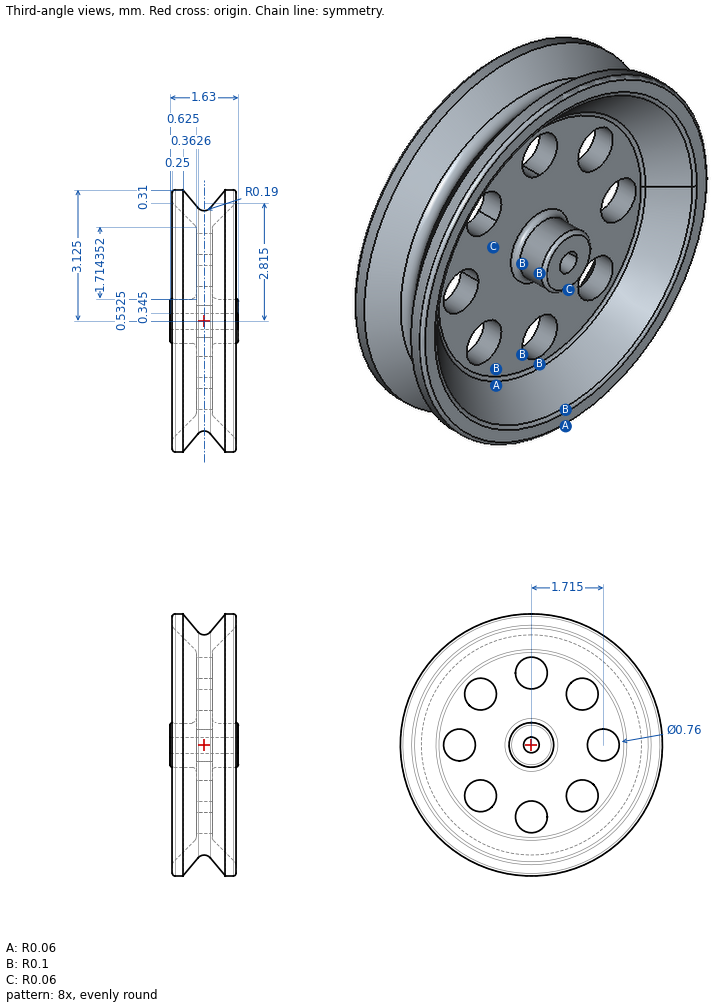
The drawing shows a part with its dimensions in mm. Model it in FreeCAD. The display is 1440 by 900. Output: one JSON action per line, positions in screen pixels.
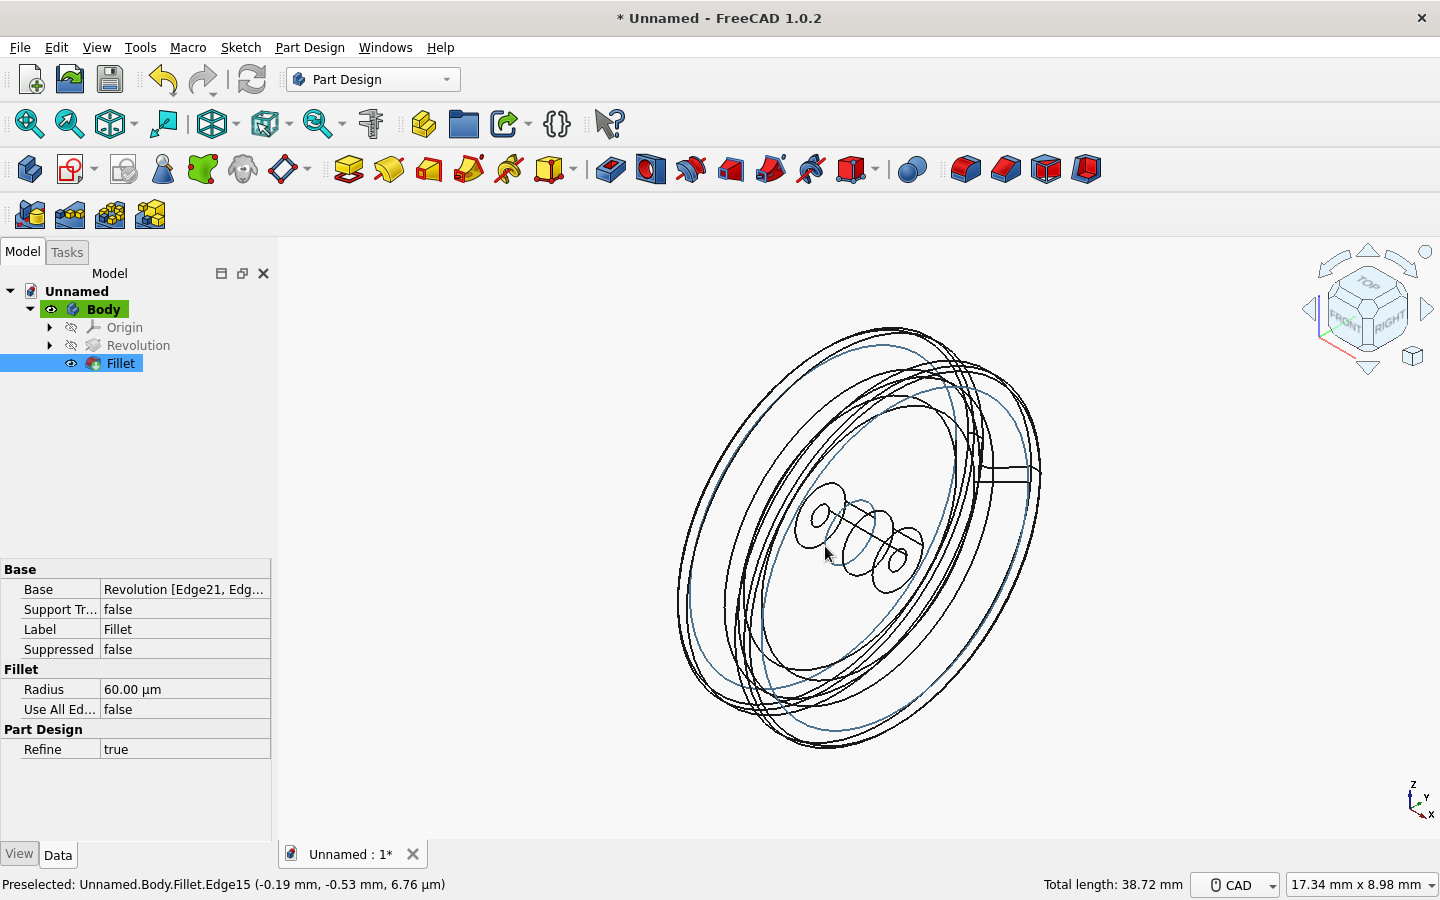
{"action": "left_click", "coordinate": [817, 668], "text": "ctrl"}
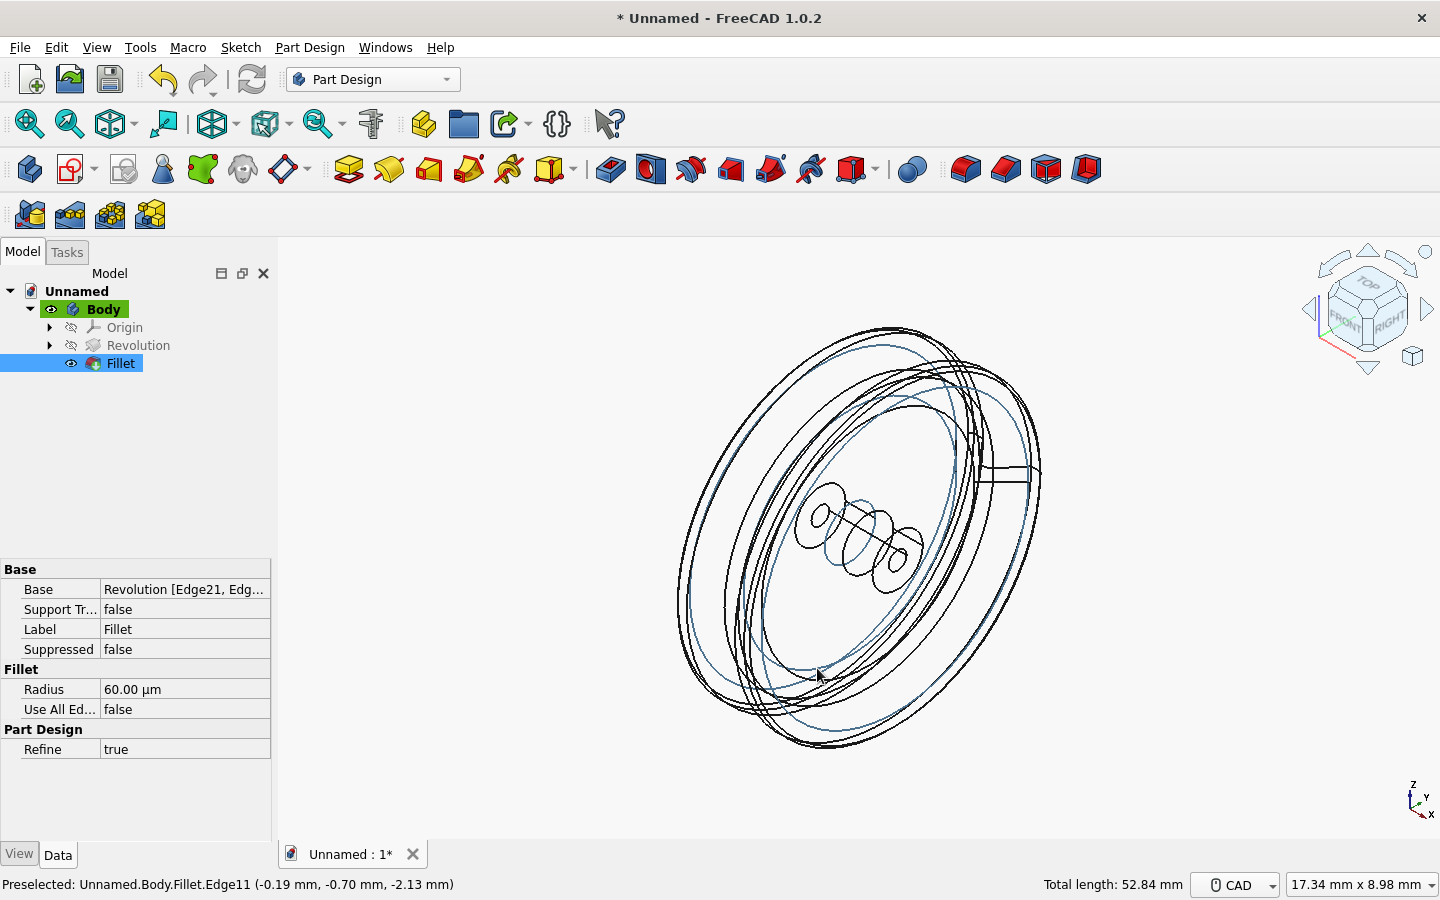
{"action": "left_click", "coordinate": [782, 664], "text": "ctrl"}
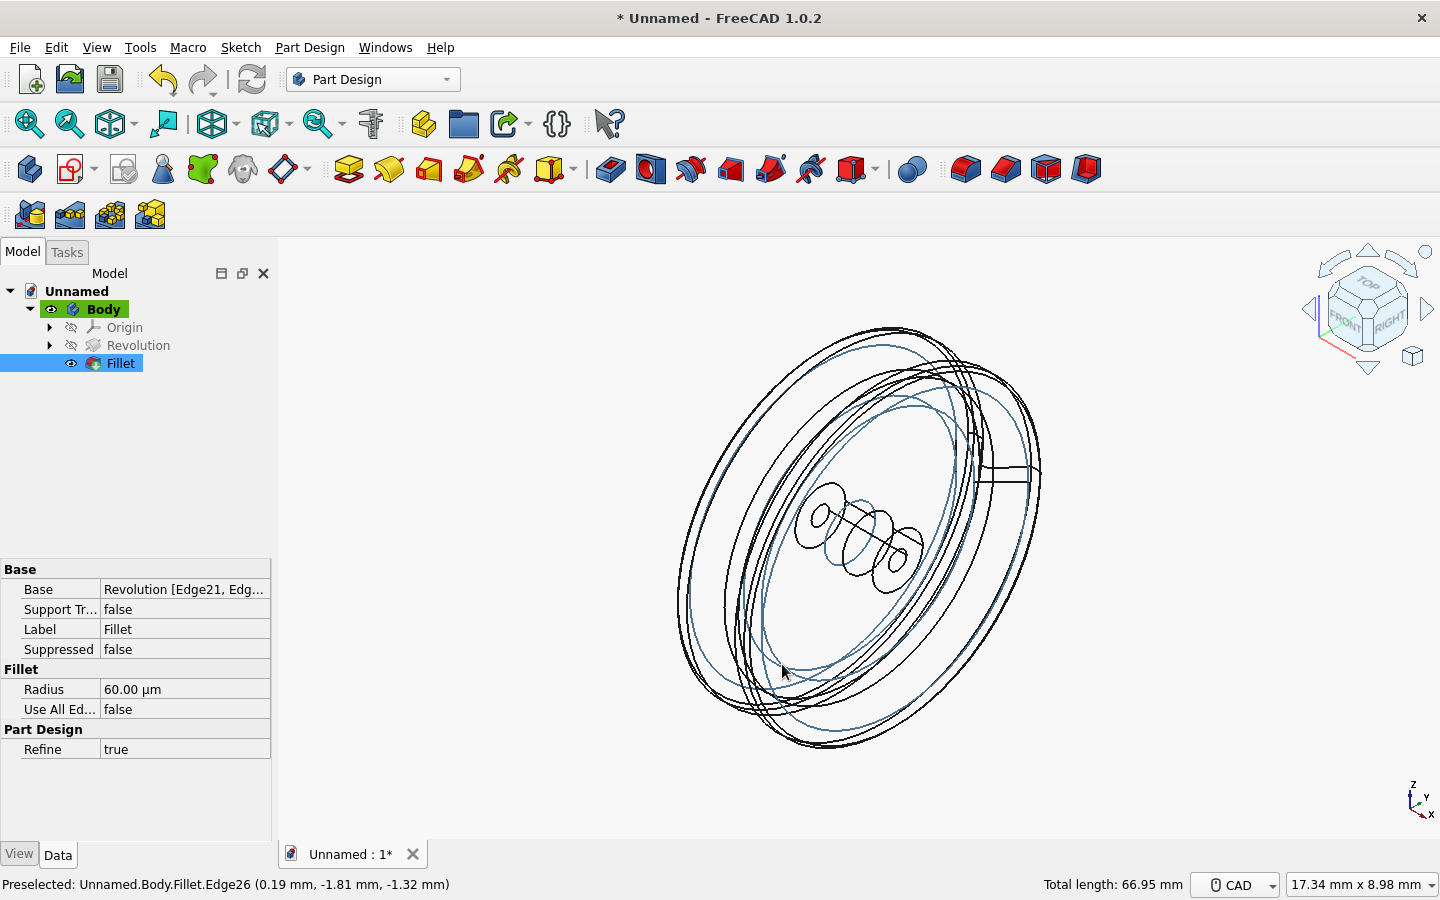
{"action": "left_click", "coordinate": [843, 557], "text": "ctrl"}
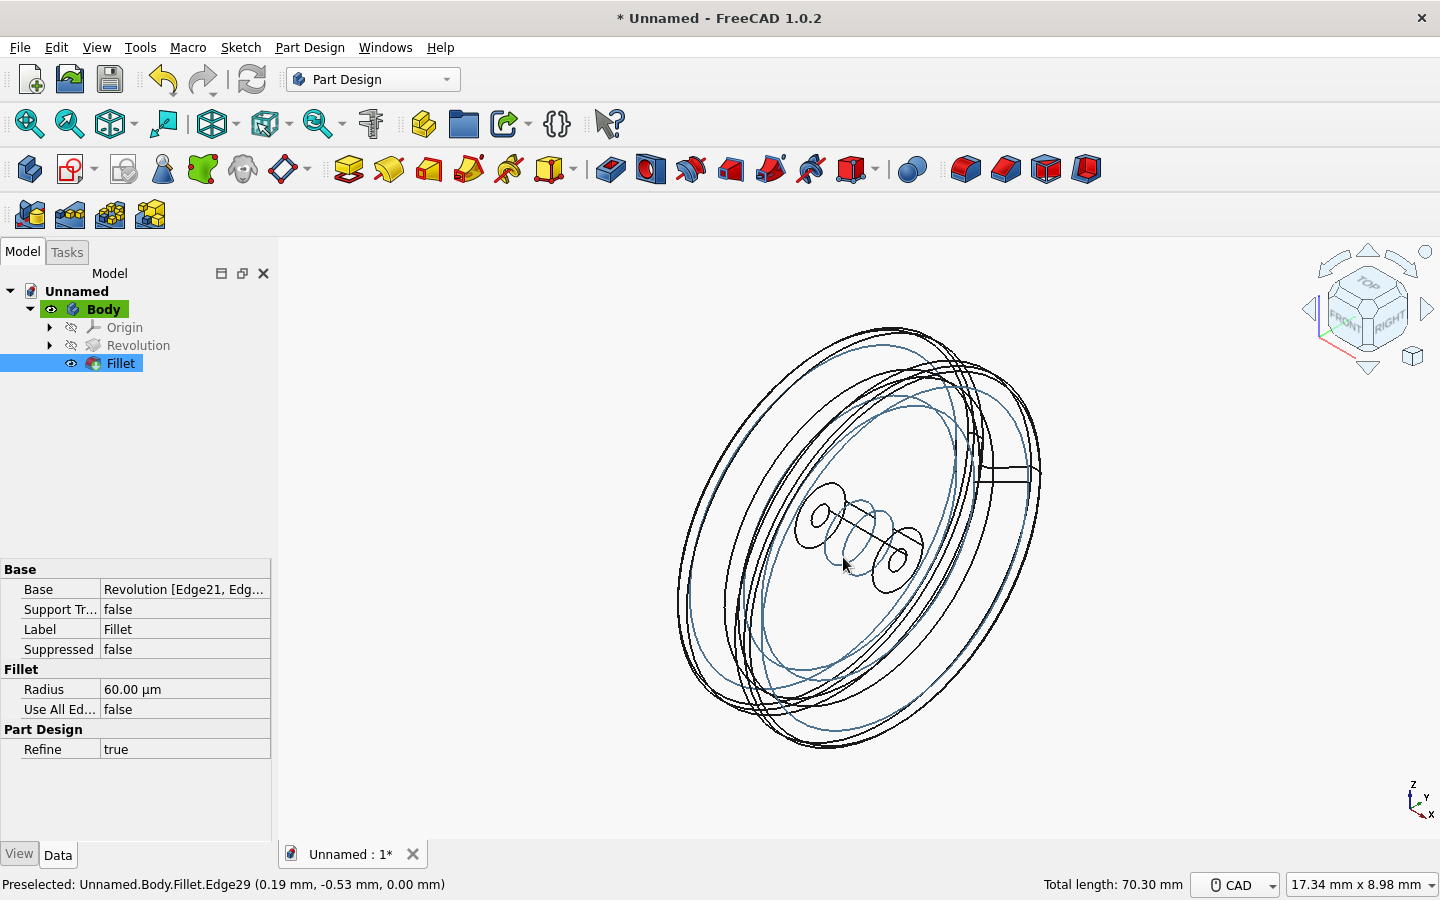
{"action": "key", "text": "v 1"}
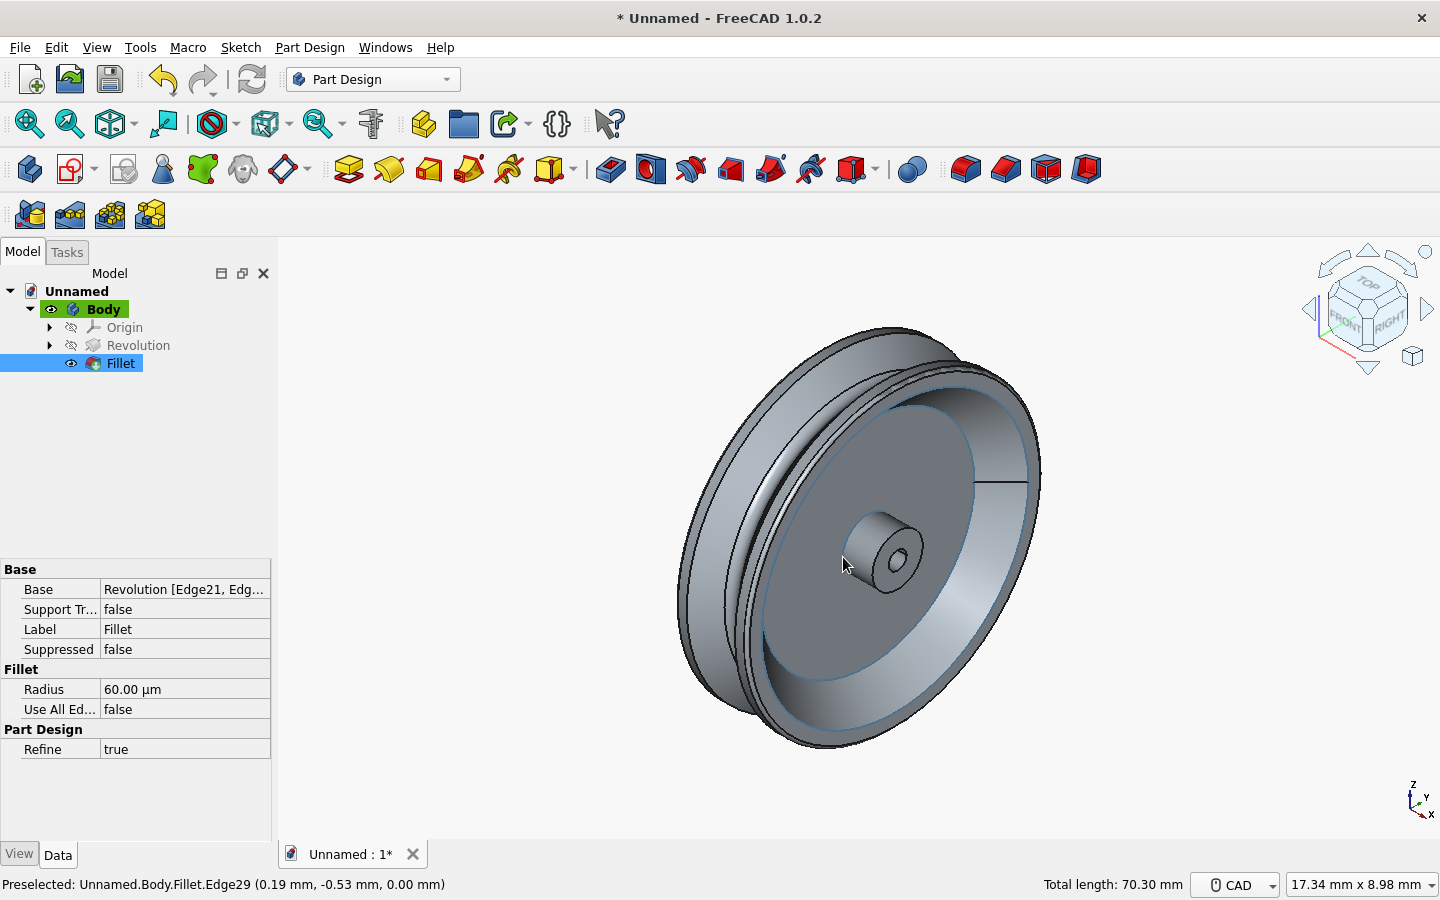
{"action": "left_click", "coordinate": [966, 170]}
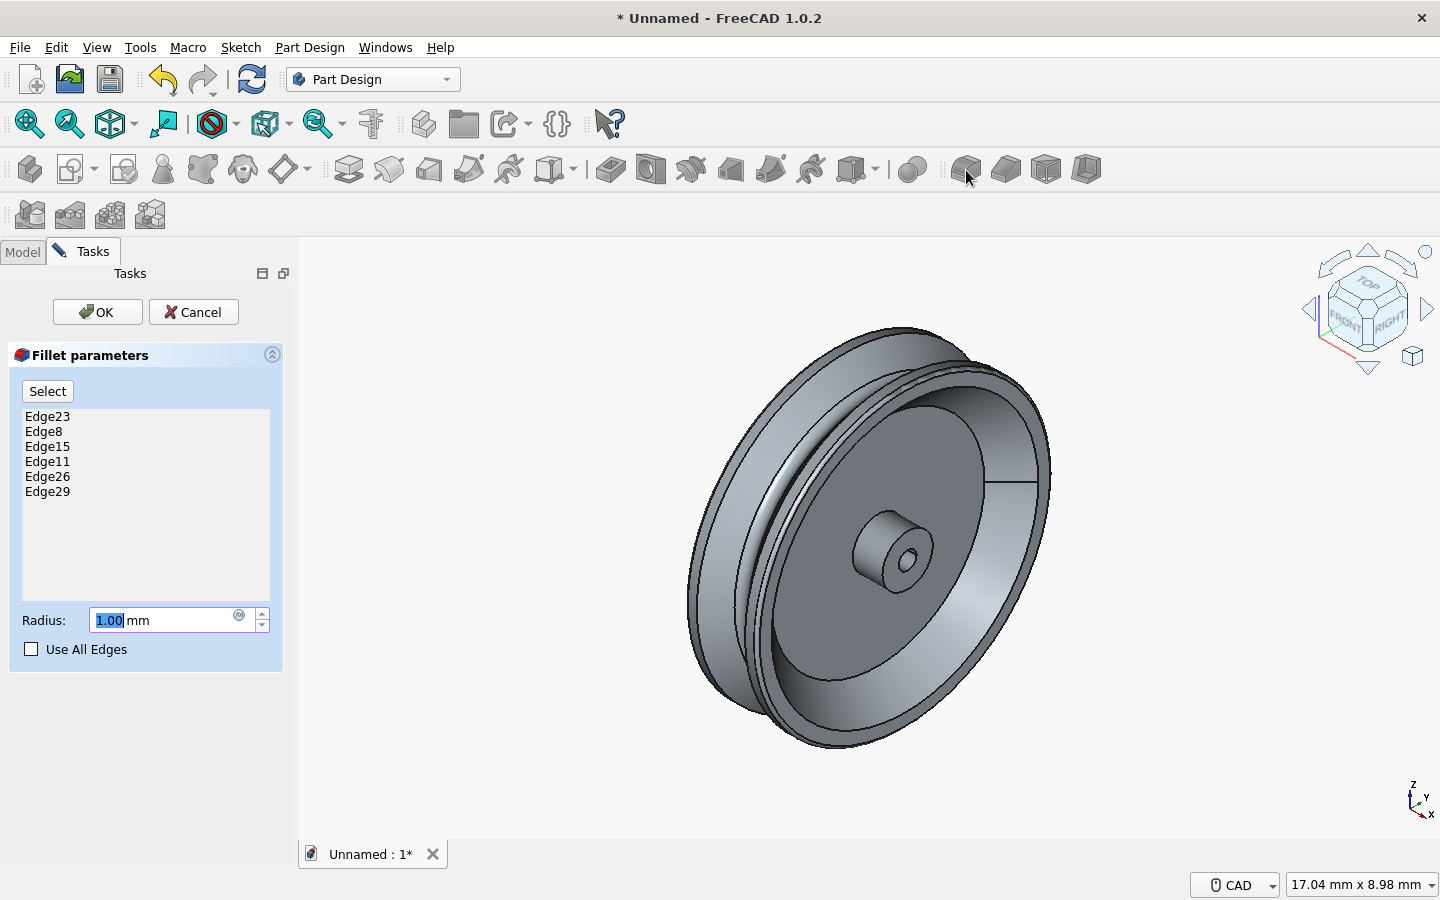
{"action": "type", "text": "0.1"}
{"action": "key", "text": "Tab"}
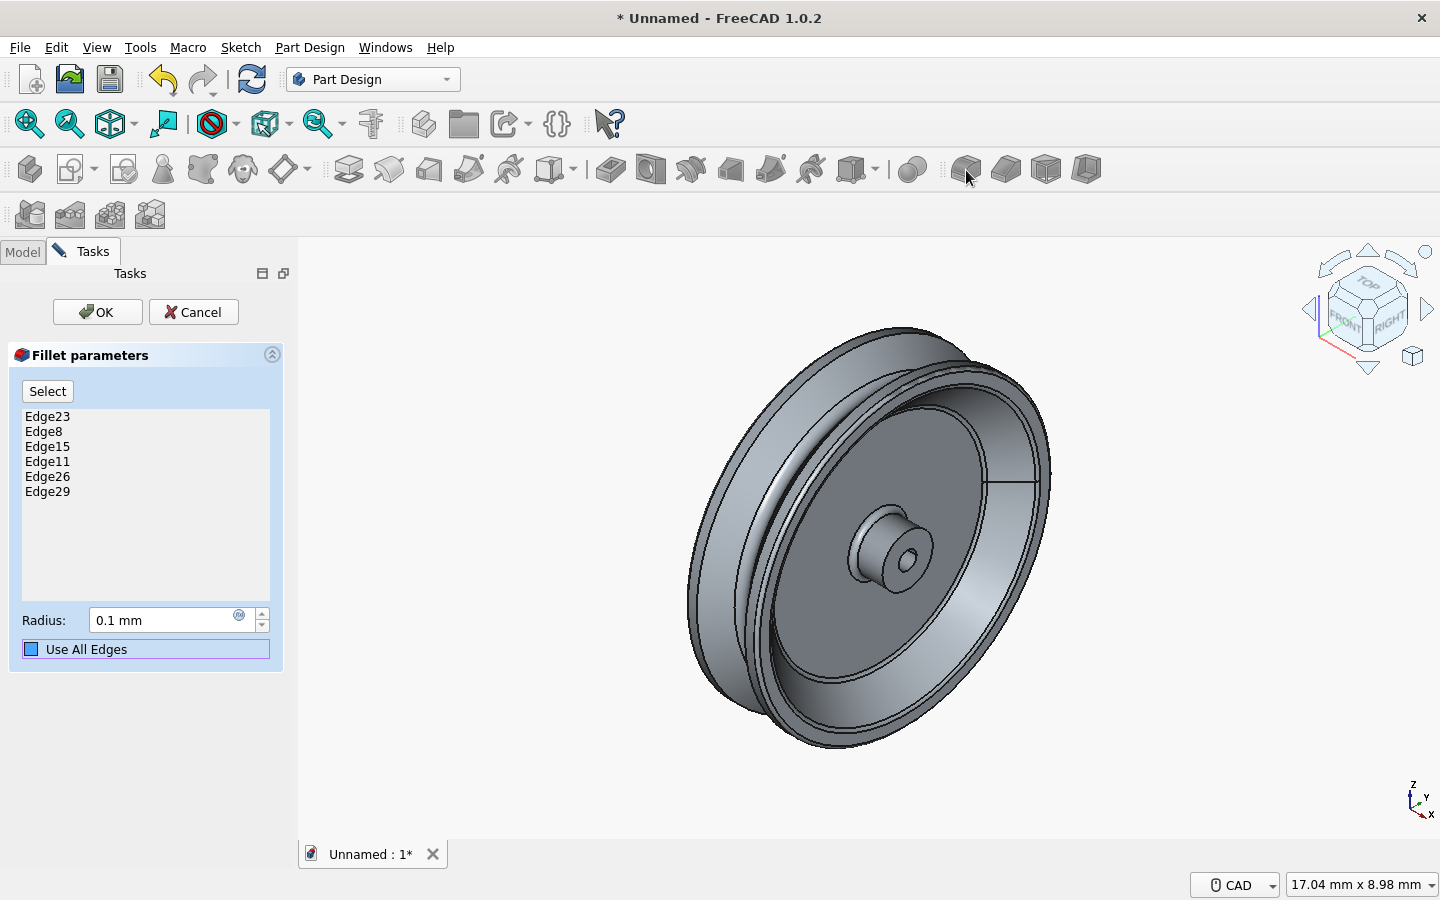
{"action": "left_click", "coordinate": [98, 312]}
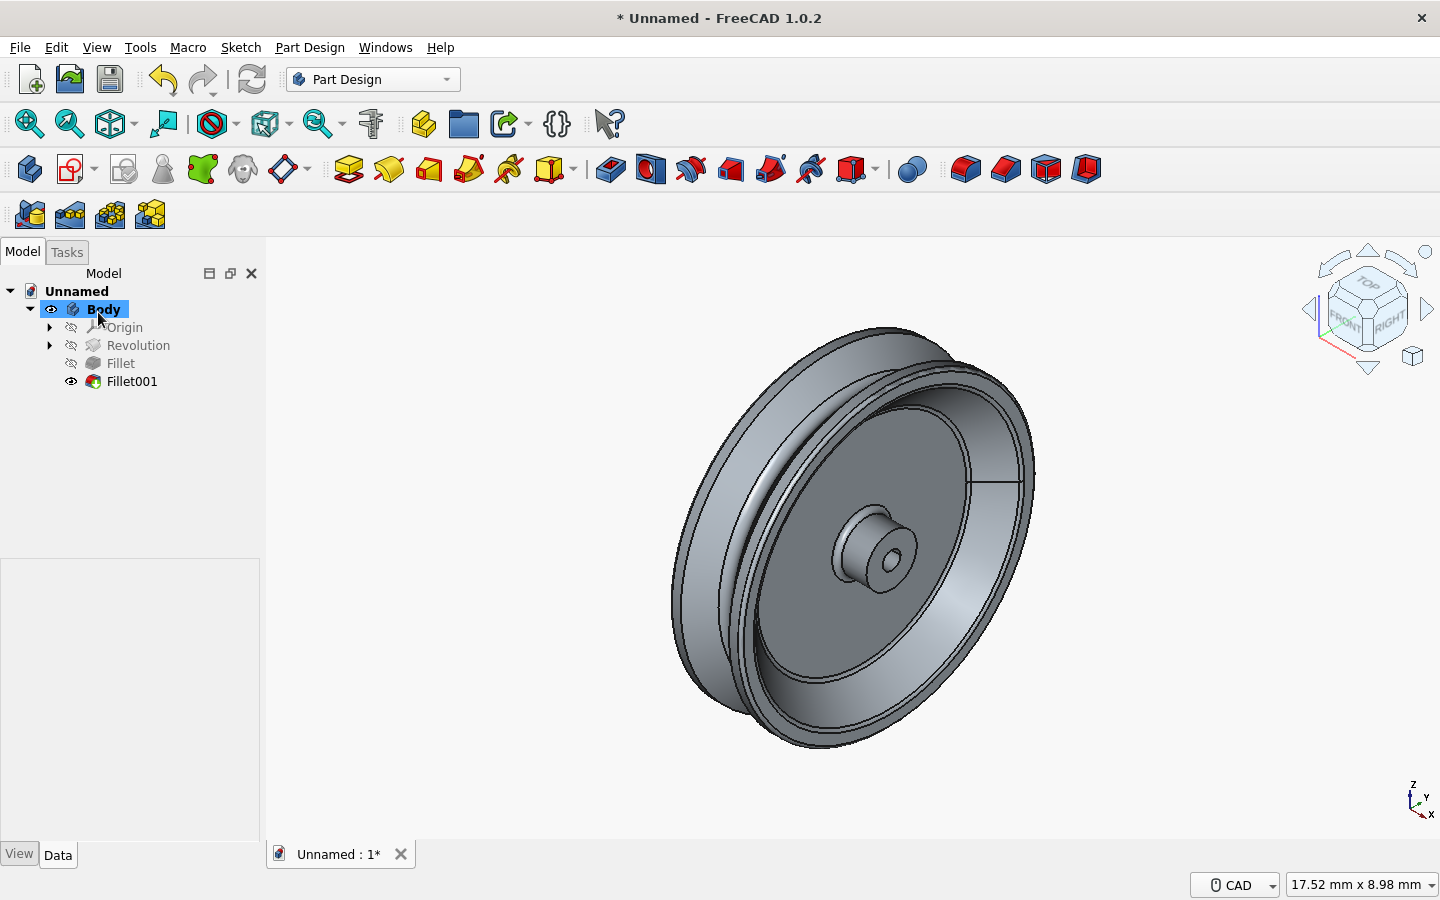
{"action": "left_click", "coordinate": [866, 574]}